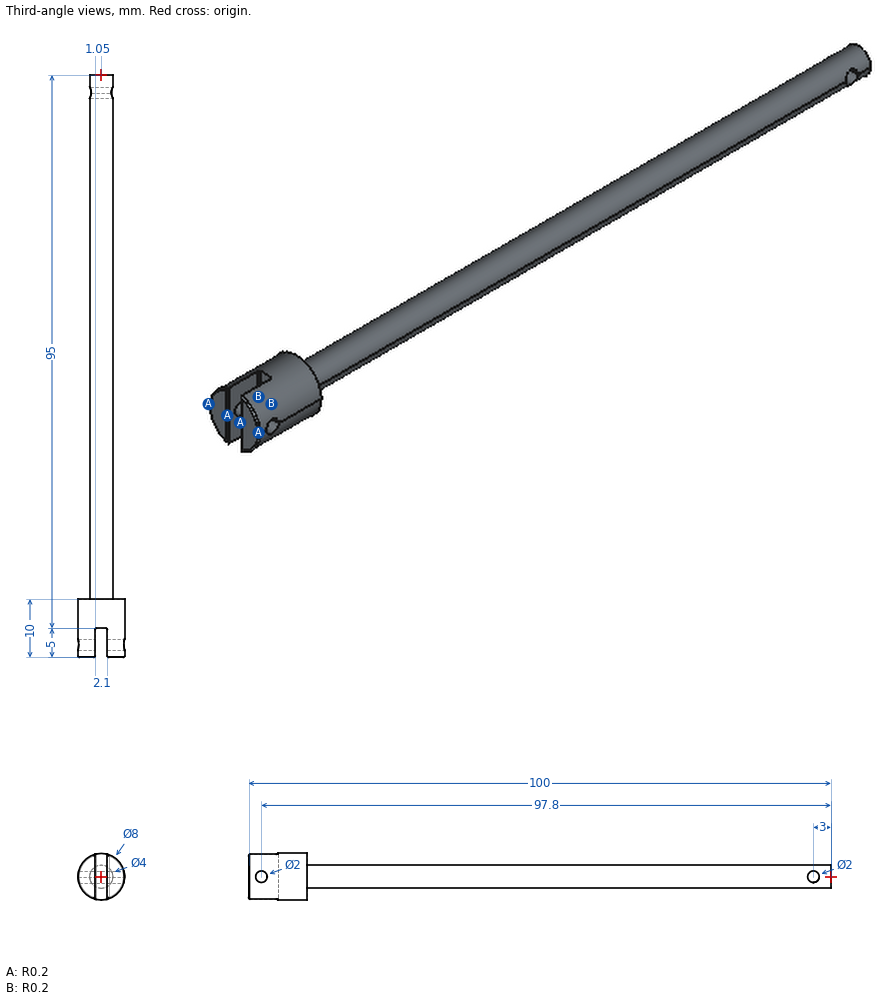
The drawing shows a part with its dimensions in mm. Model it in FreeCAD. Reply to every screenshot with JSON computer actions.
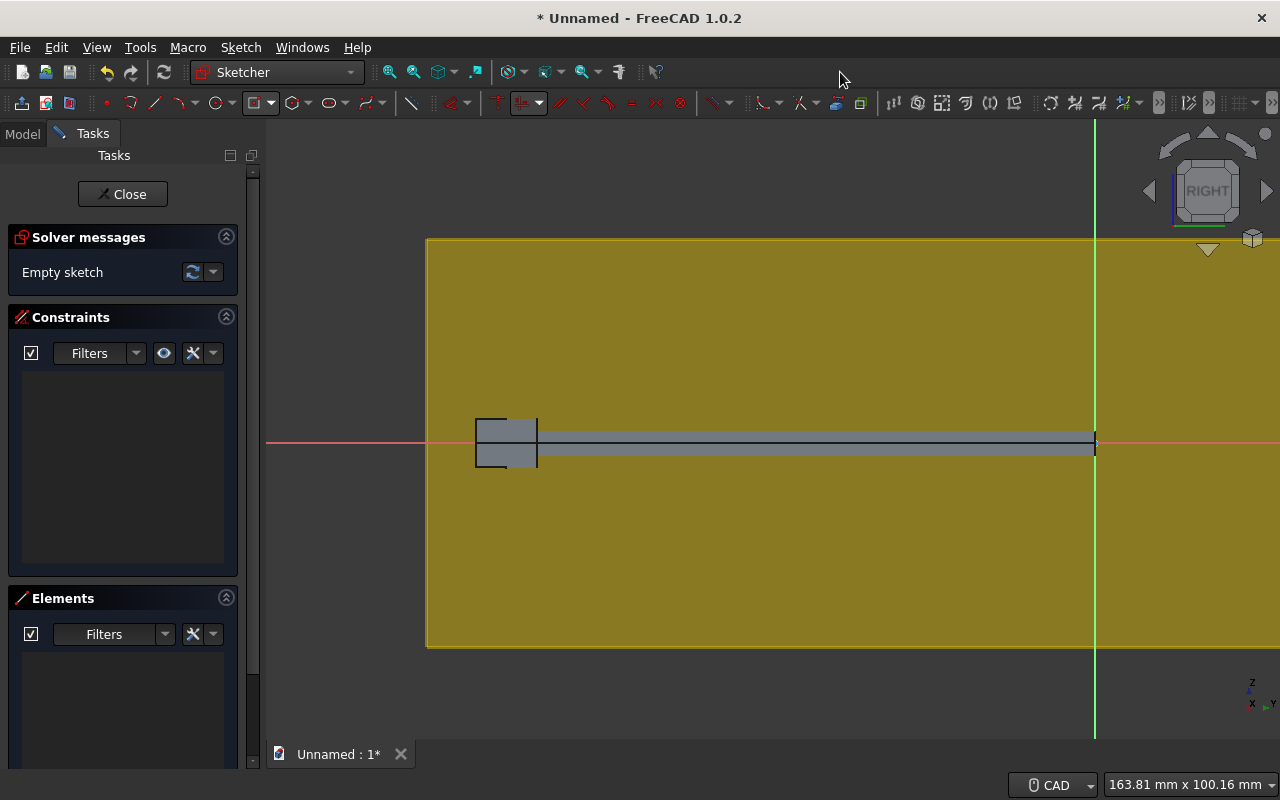
{"action": "left_click", "coordinate": [70, 104]}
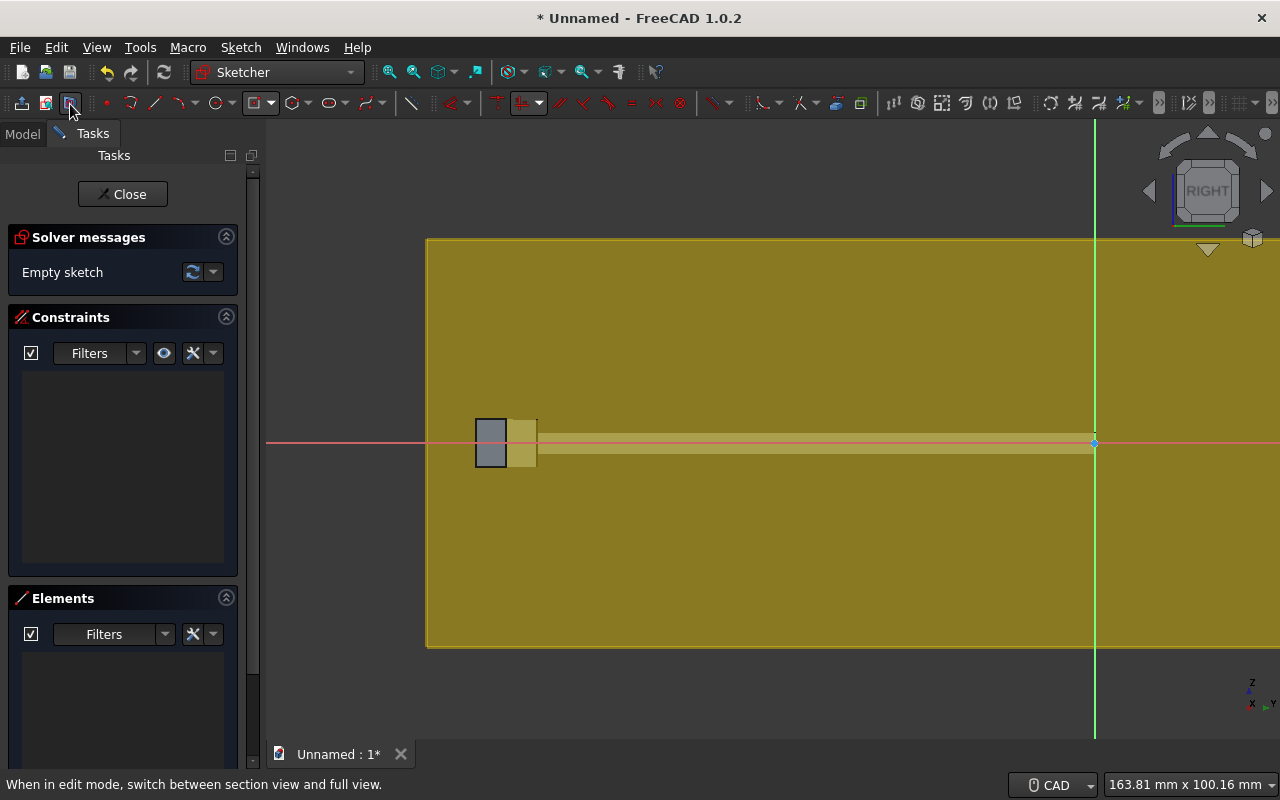
{"action": "scroll", "coordinate": [478, 444], "scroll_direction": "up", "scroll_amount": 15}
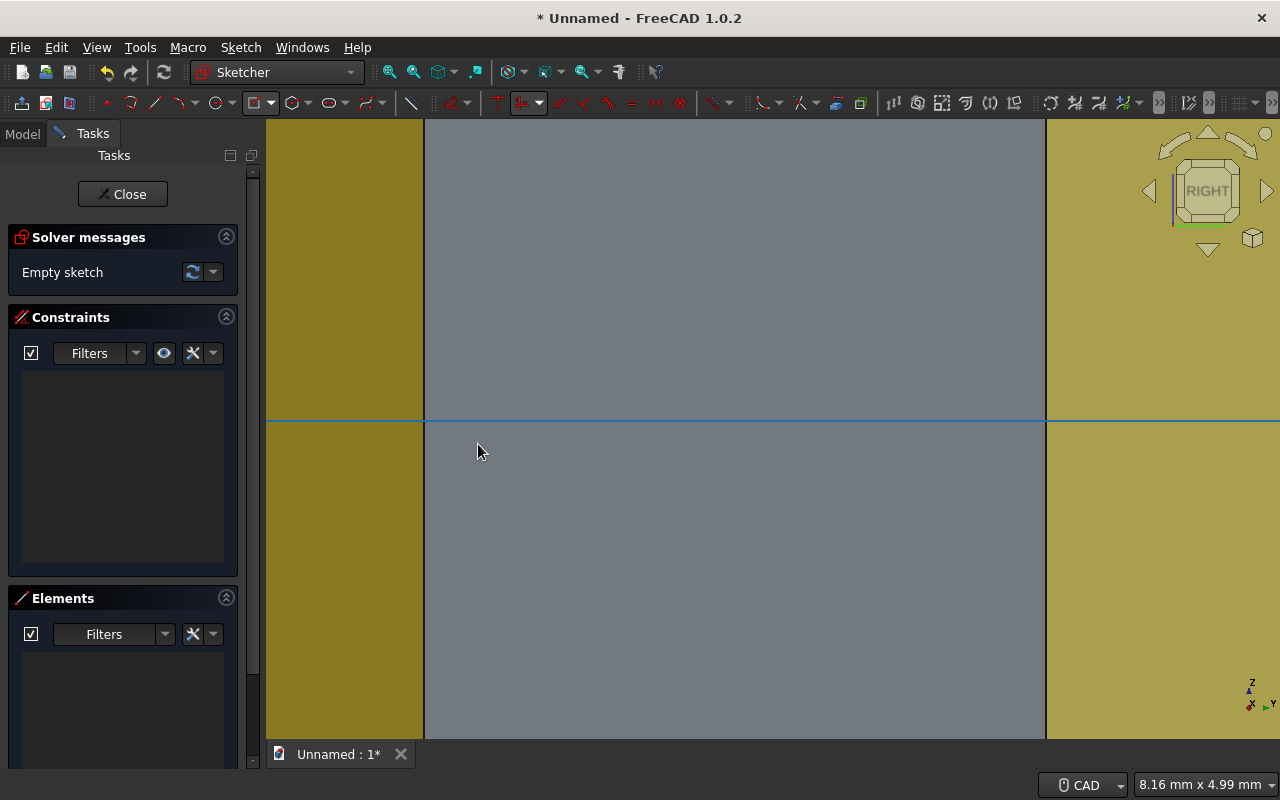
{"action": "scroll", "coordinate": [685, 405], "scroll_direction": "up", "scroll_amount": 2}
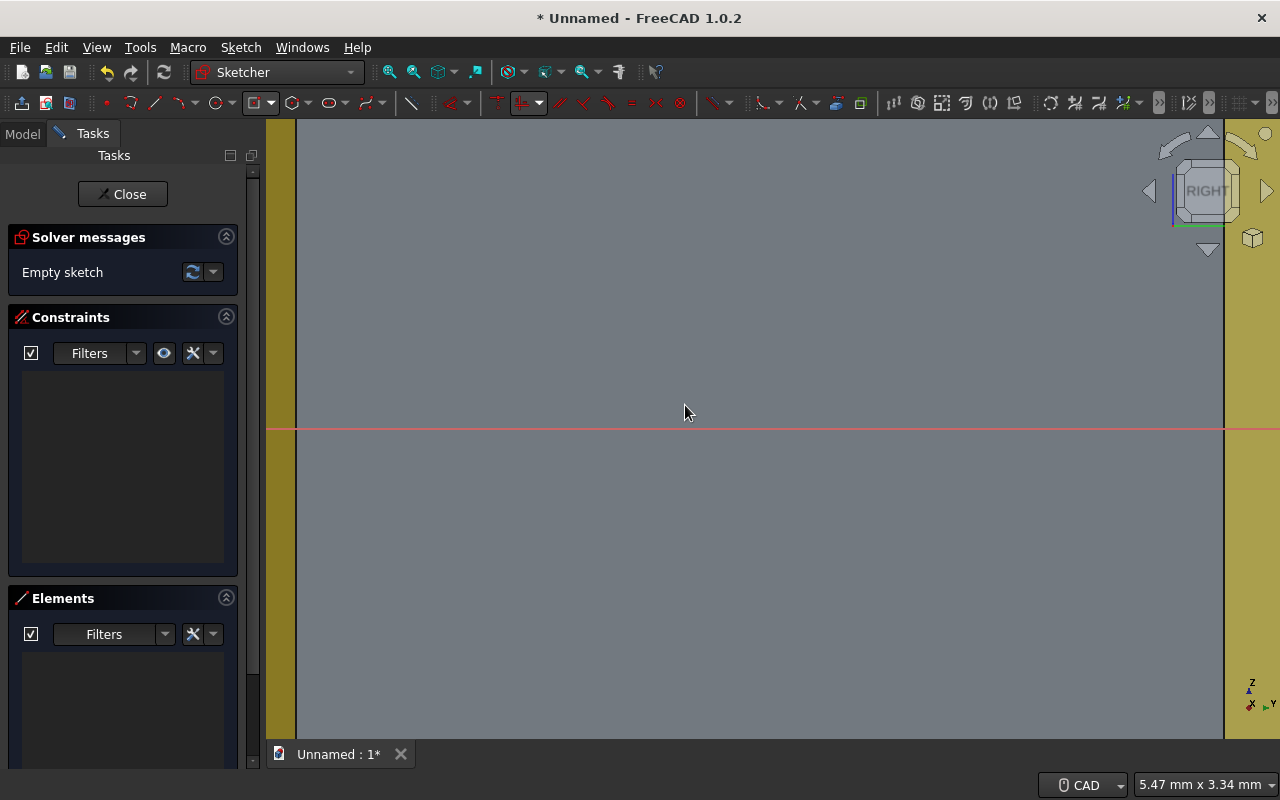
{"action": "left_click", "coordinate": [216, 104]}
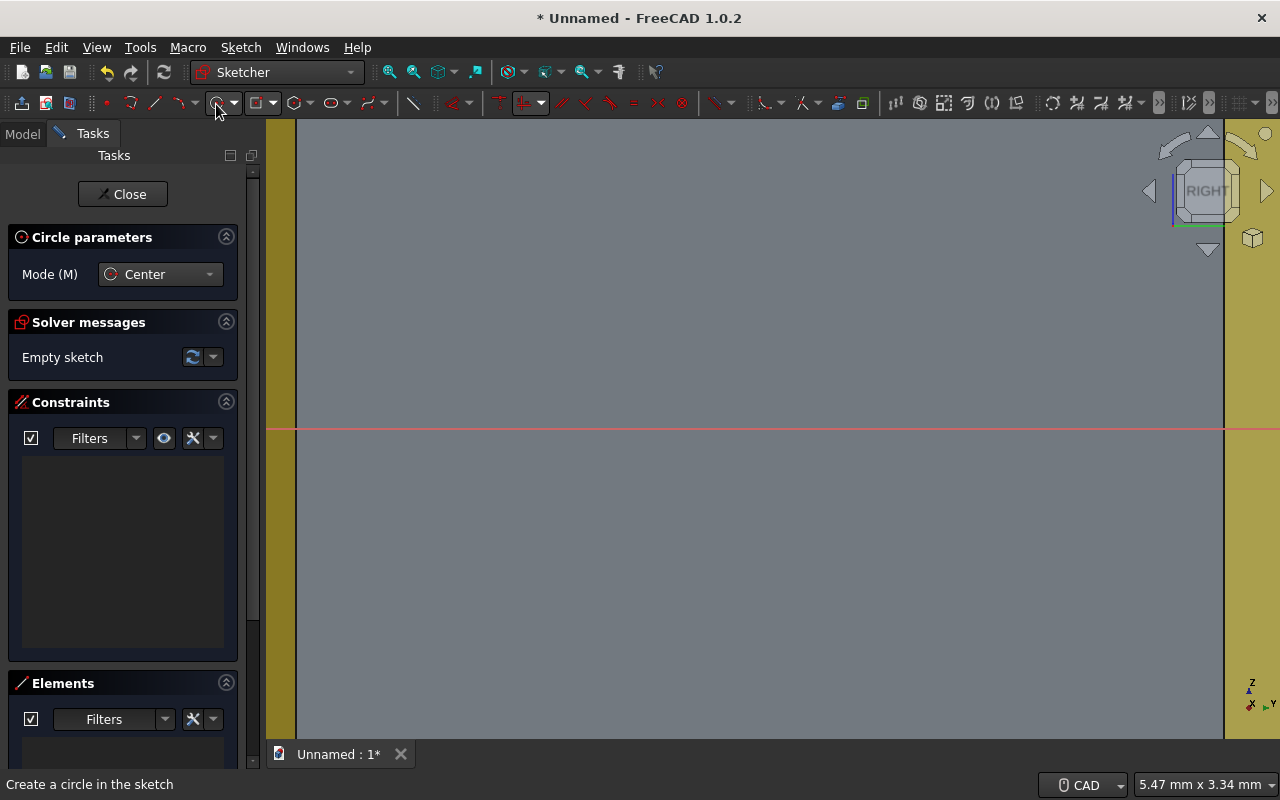
{"action": "left_click", "coordinate": [704, 429]}
{"action": "left_click", "coordinate": [835, 298]}
{"action": "key", "text": "Escape"}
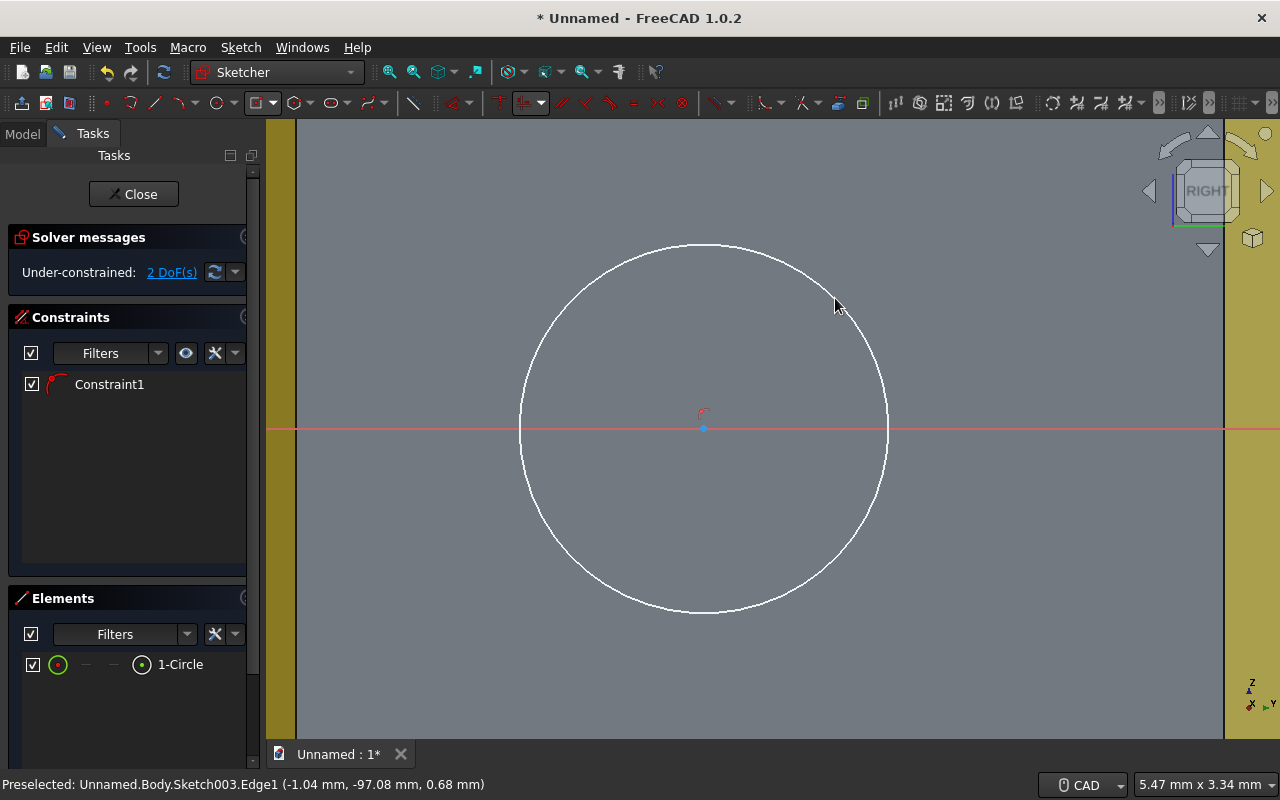
{"action": "key", "text": "d"}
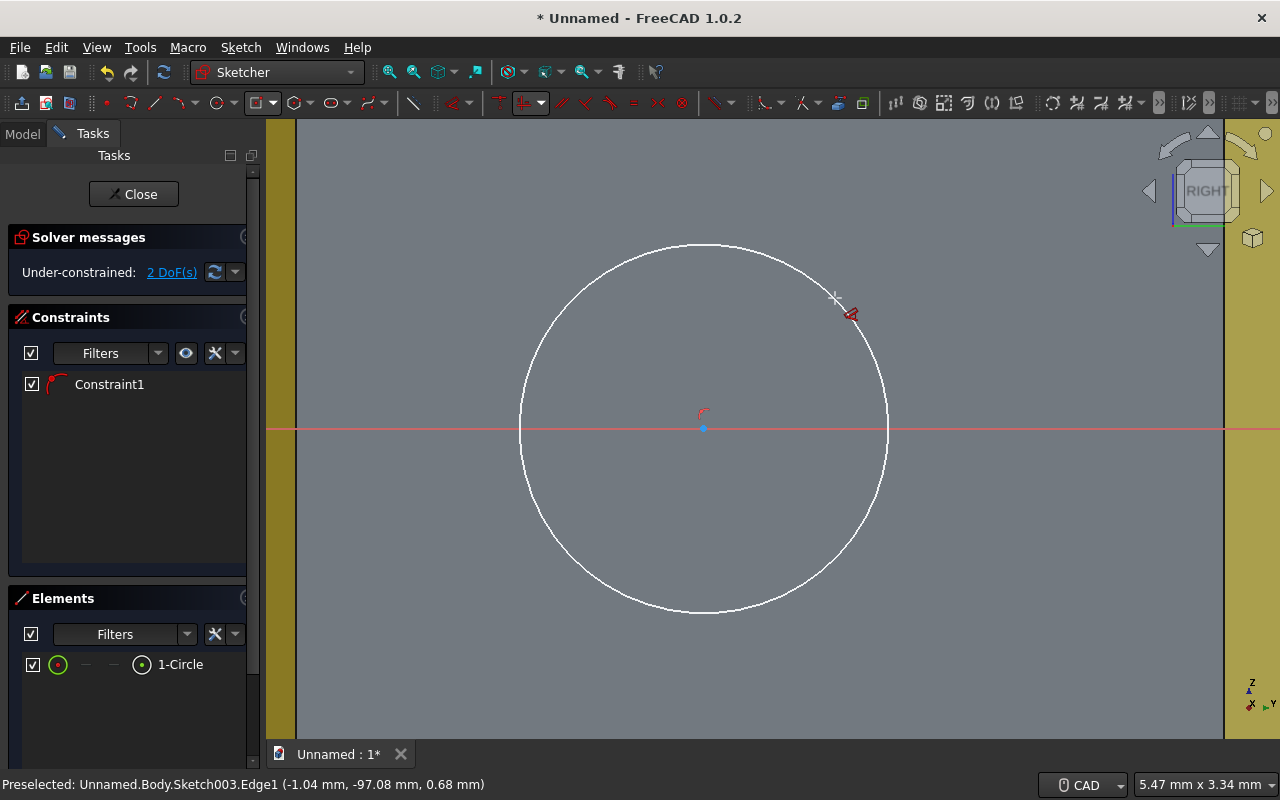
{"action": "left_click", "coordinate": [834, 298]}
{"action": "left_click", "coordinate": [857, 275]}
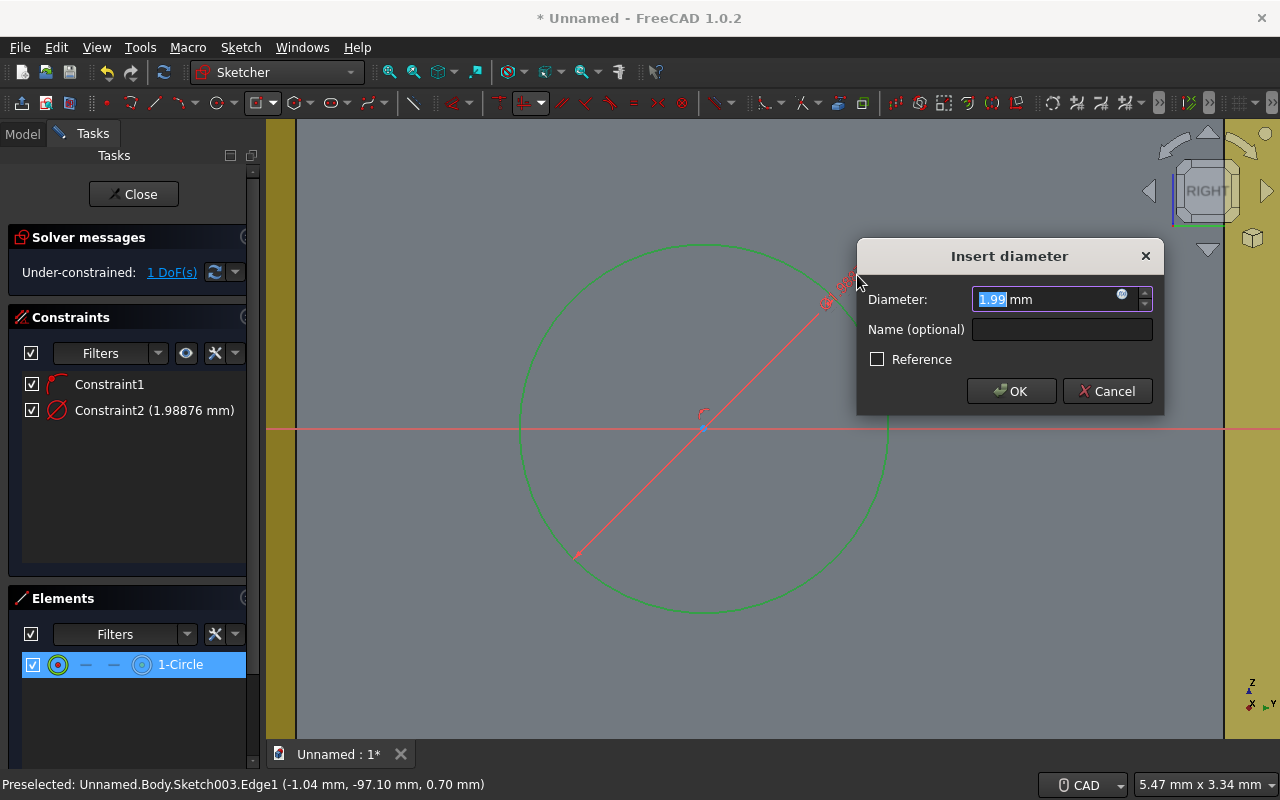
{"action": "type", "text": "2"}
{"action": "key", "text": "Return"}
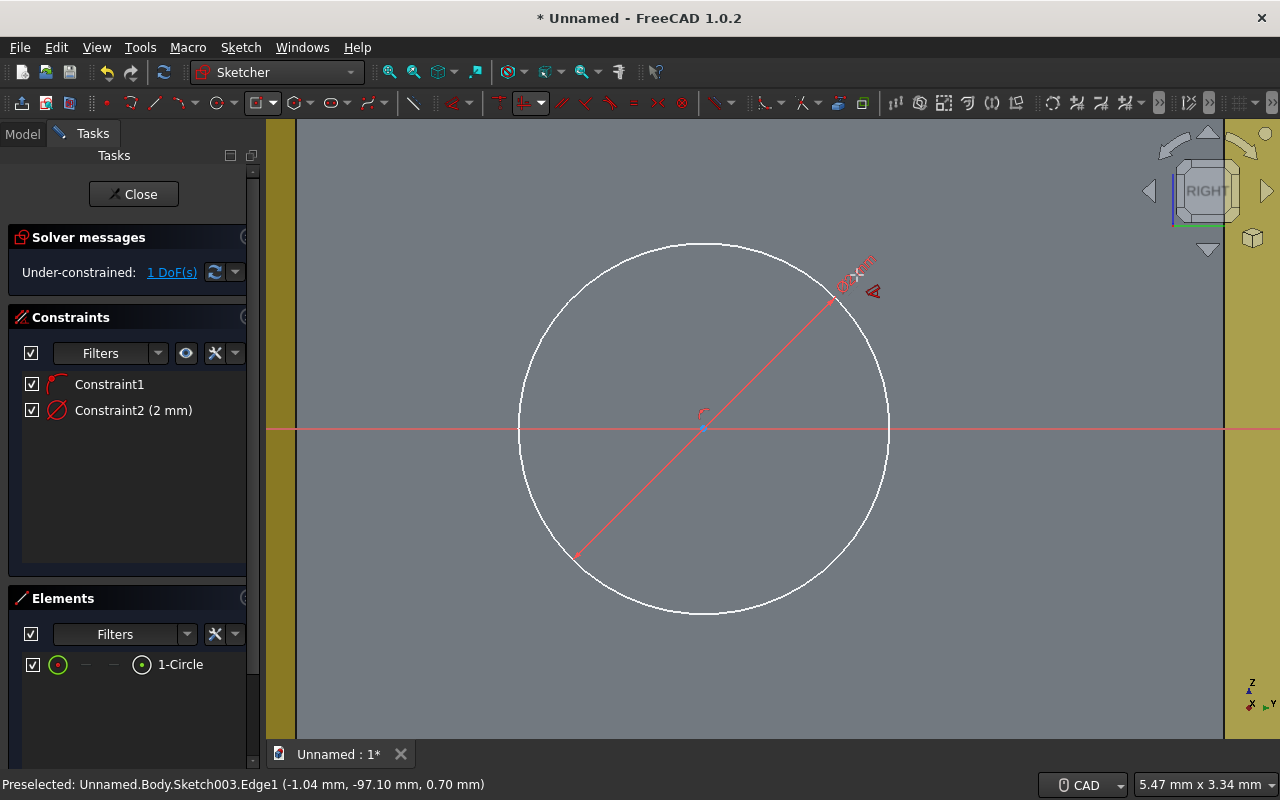
{"action": "left_click", "coordinate": [704, 429]}
{"action": "left_click", "coordinate": [910, 463]}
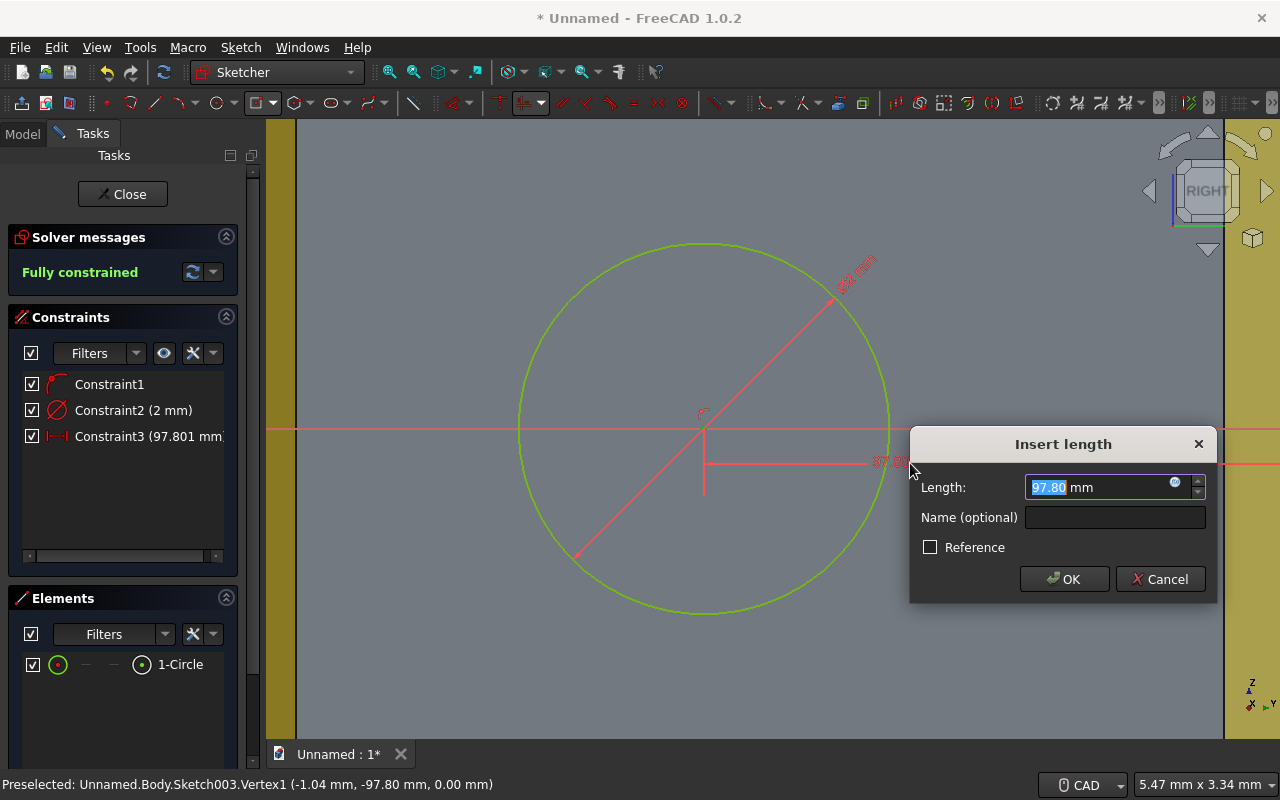
{"action": "type", "text": "97.8"}
{"action": "key", "text": "Return"}
{"action": "key", "text": "Escape"}